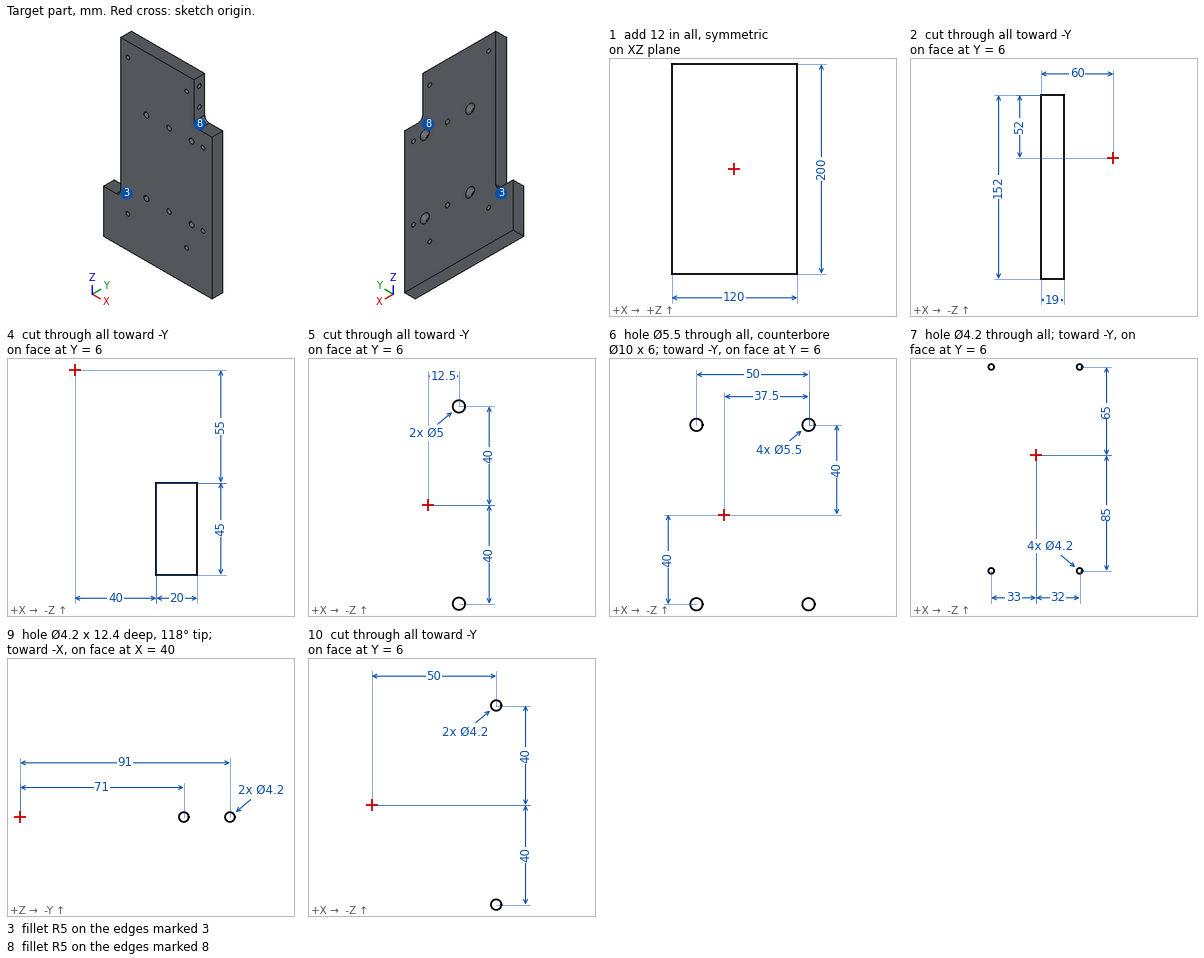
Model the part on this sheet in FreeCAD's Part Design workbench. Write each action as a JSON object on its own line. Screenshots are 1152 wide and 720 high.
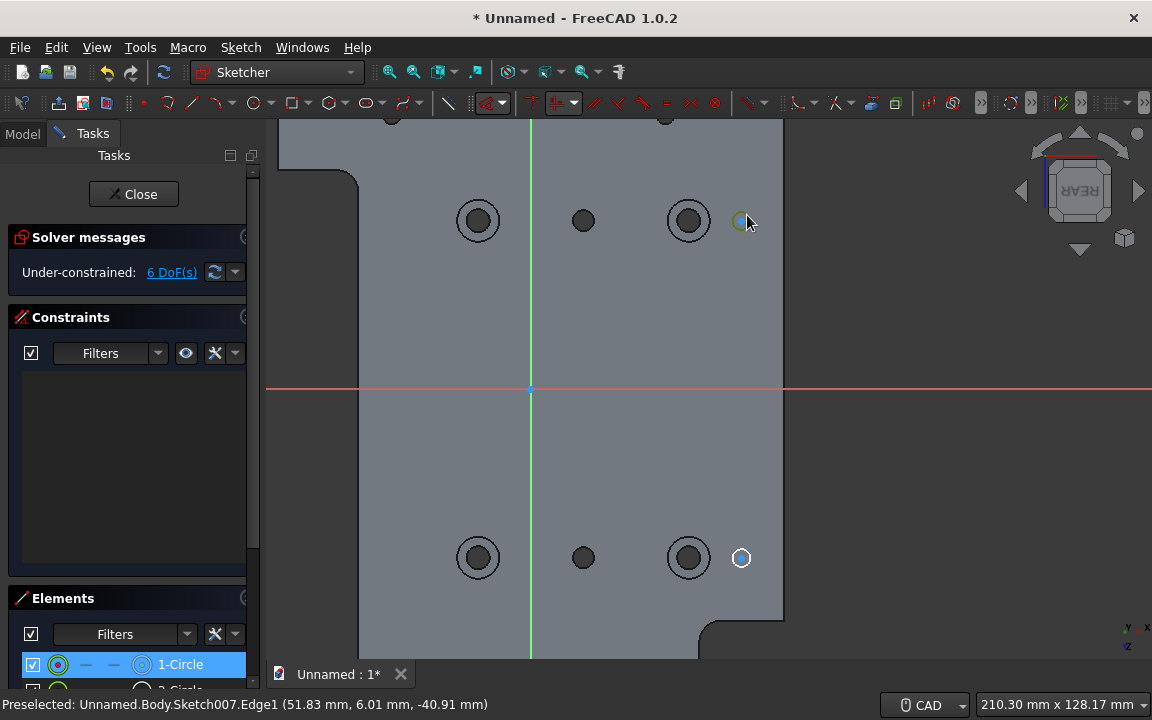
{"action": "scroll", "coordinate": [748, 552], "scroll_direction": "up", "scroll_amount": 3}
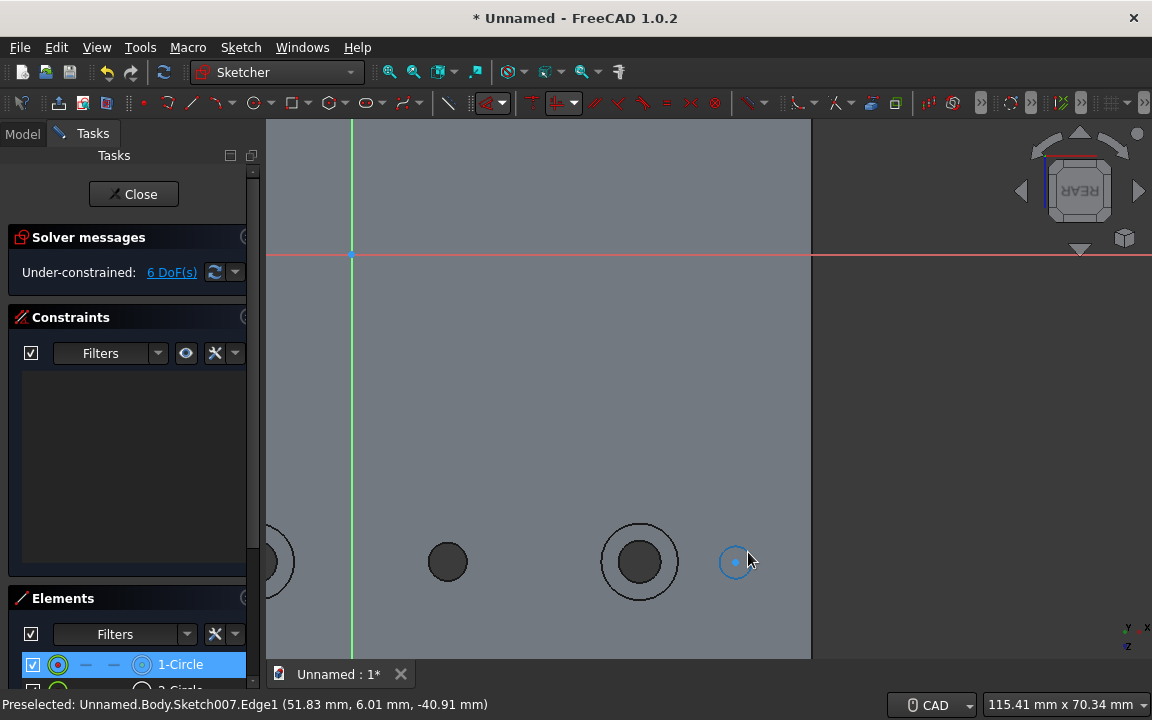
{"action": "left_click", "coordinate": [747, 551]}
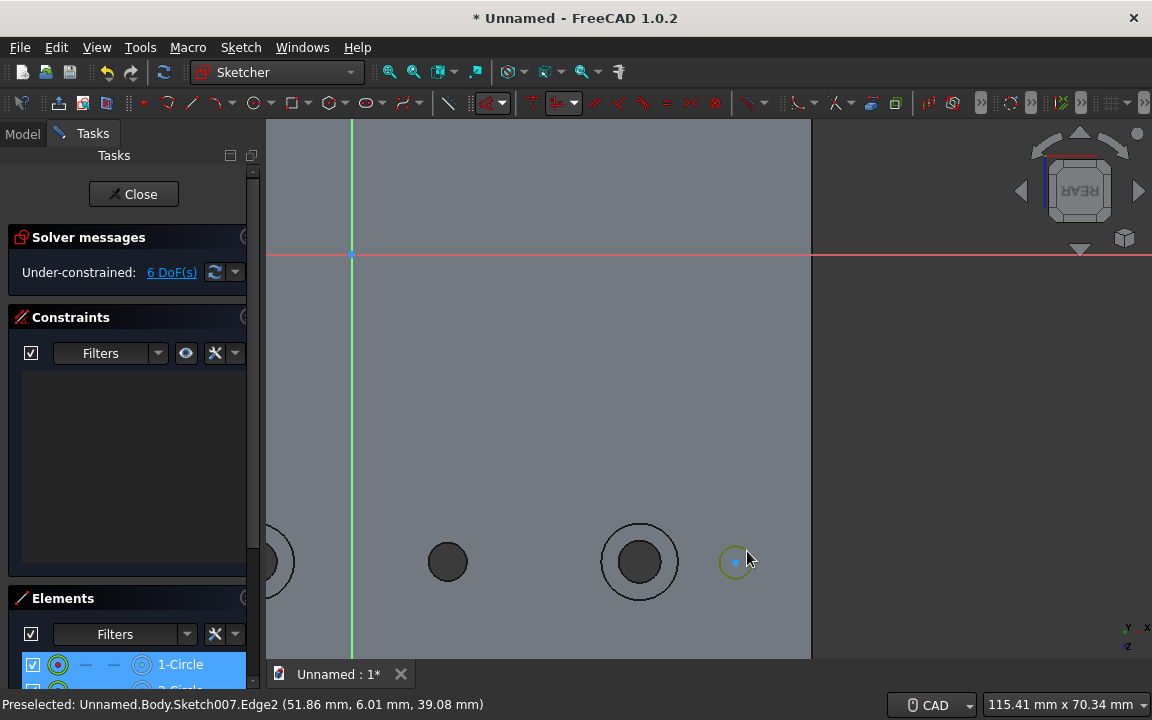
{"action": "left_click", "coordinate": [668, 104]}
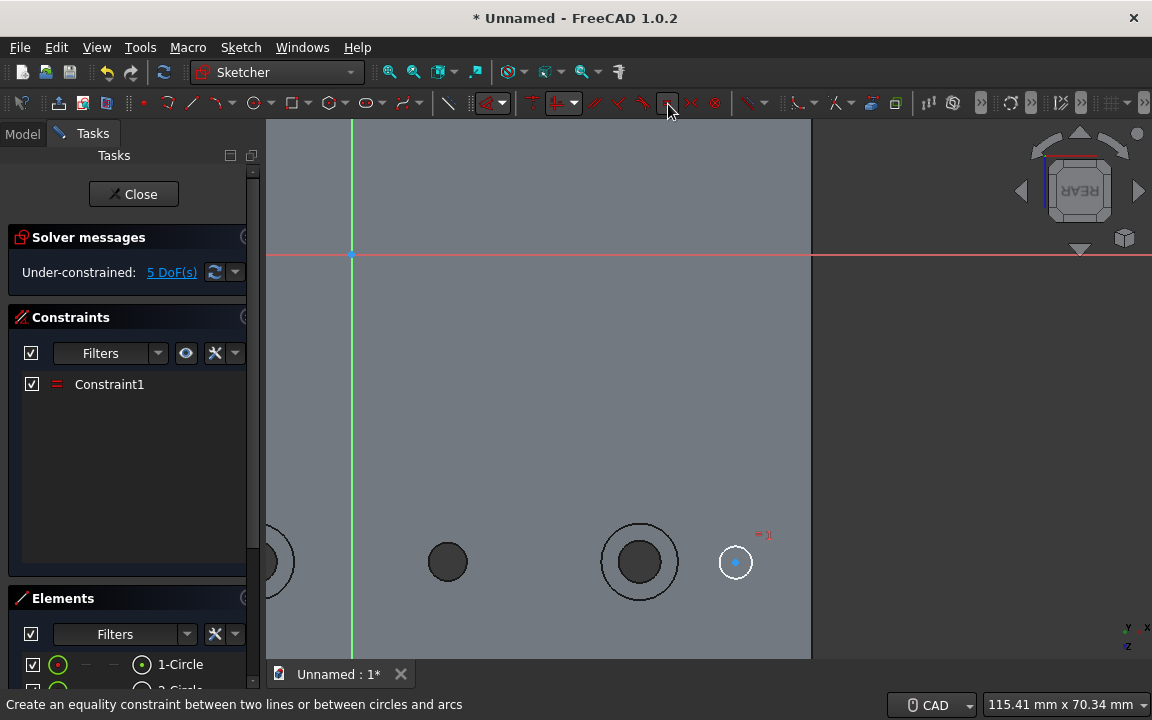
{"action": "scroll", "coordinate": [748, 552], "scroll_direction": "down", "scroll_amount": 3}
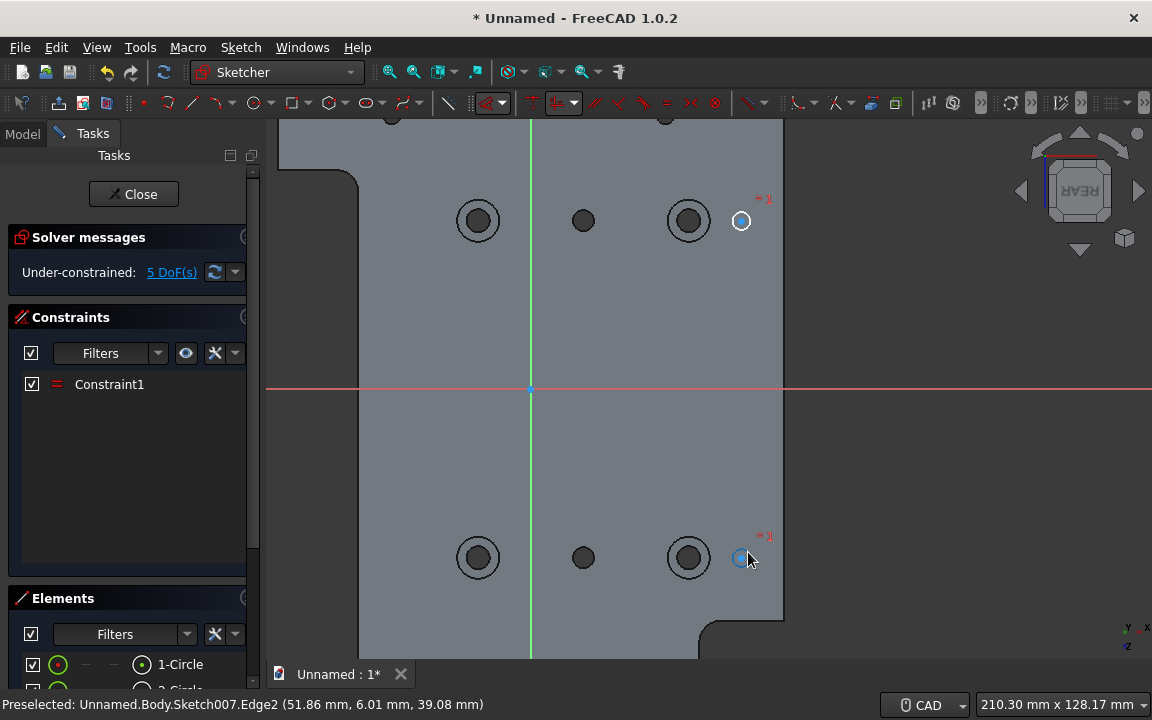
{"action": "left_click", "coordinate": [741, 221]}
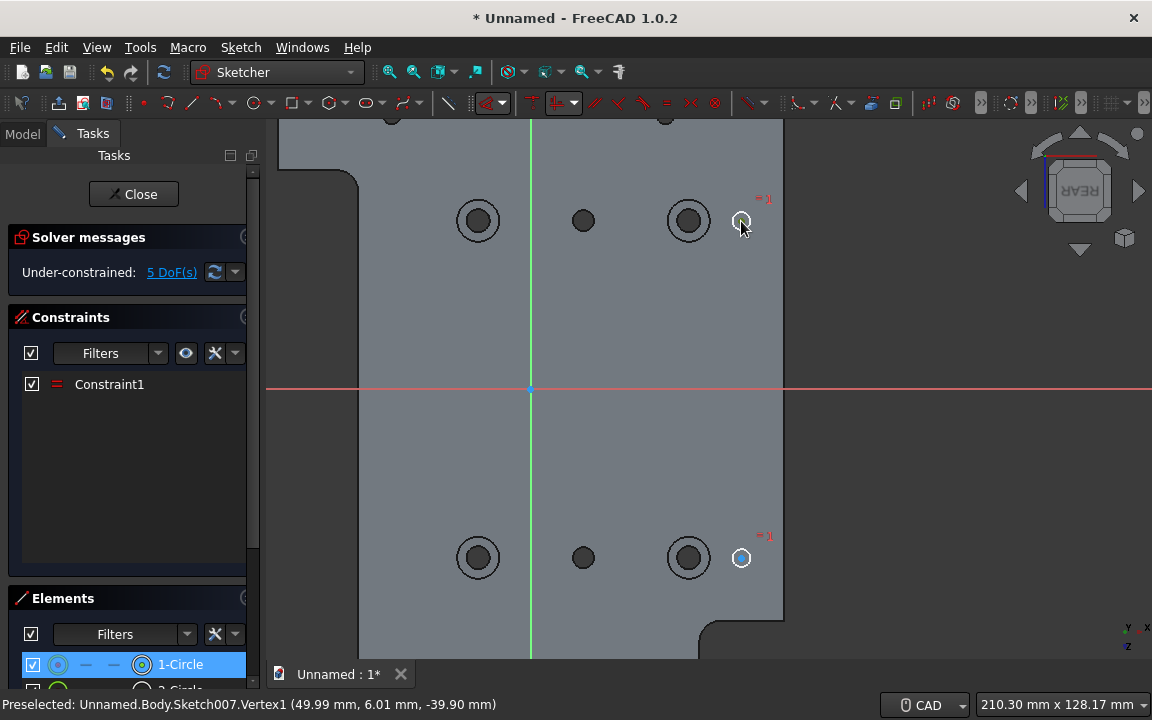
{"action": "left_click", "coordinate": [742, 558]}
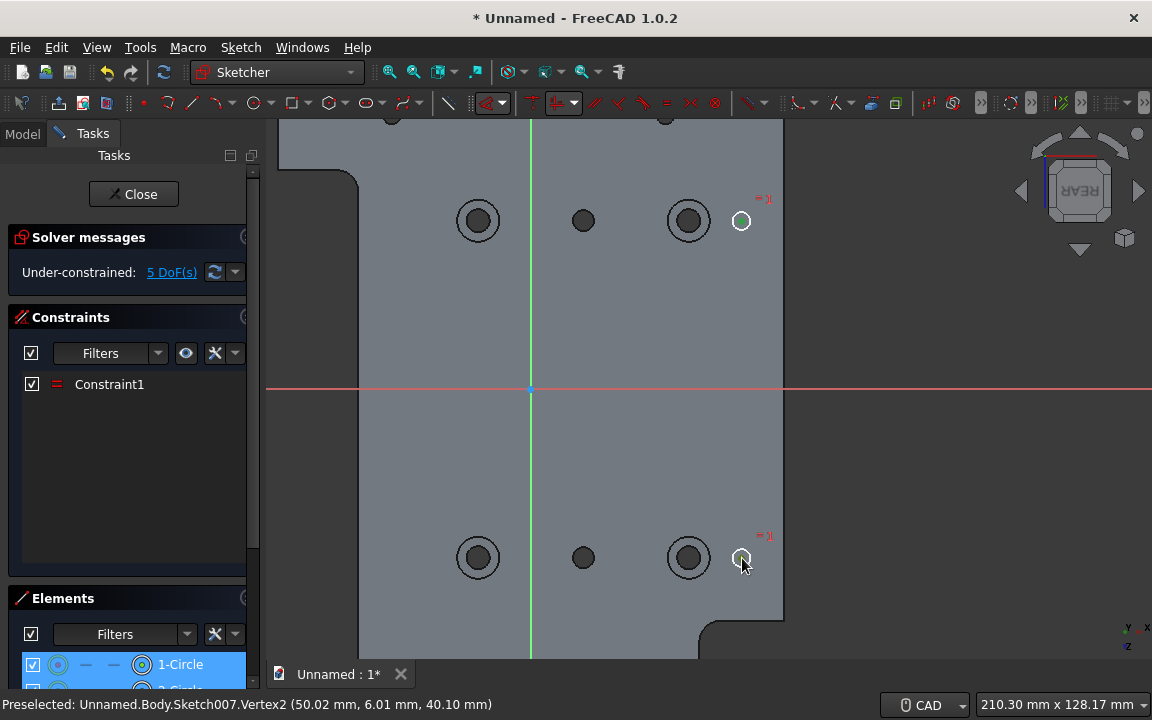
{"action": "key", "text": "v"}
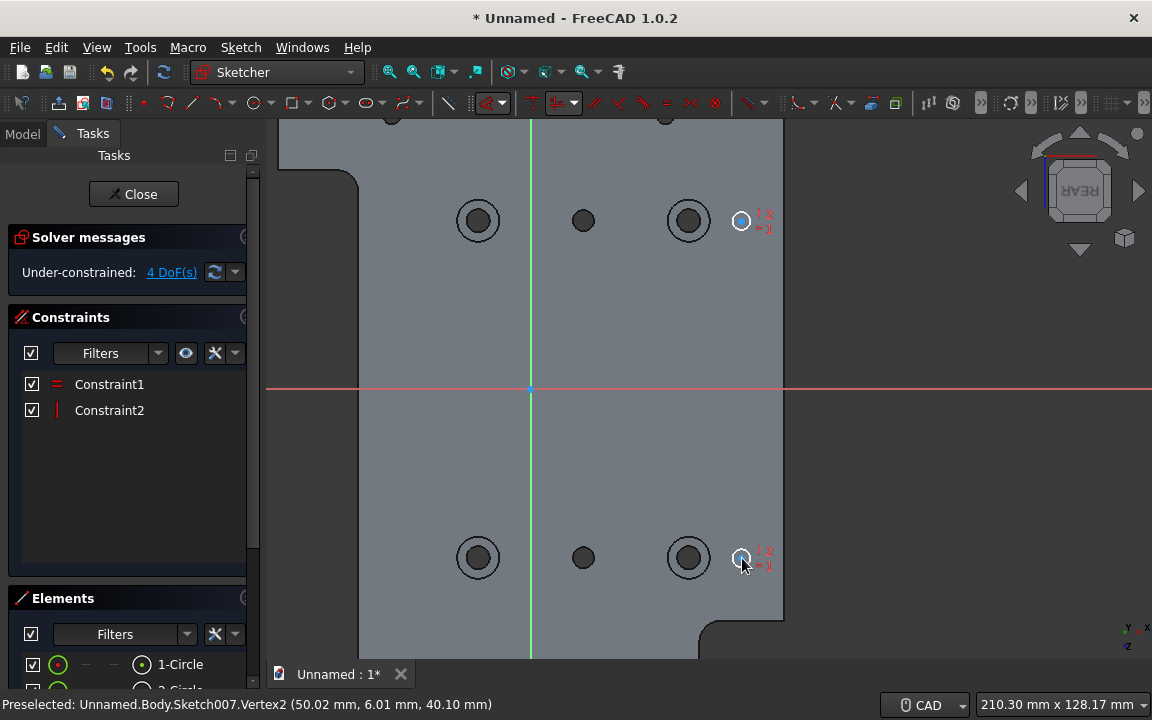
{"action": "scroll", "coordinate": [742, 212], "scroll_direction": "up", "scroll_amount": 5}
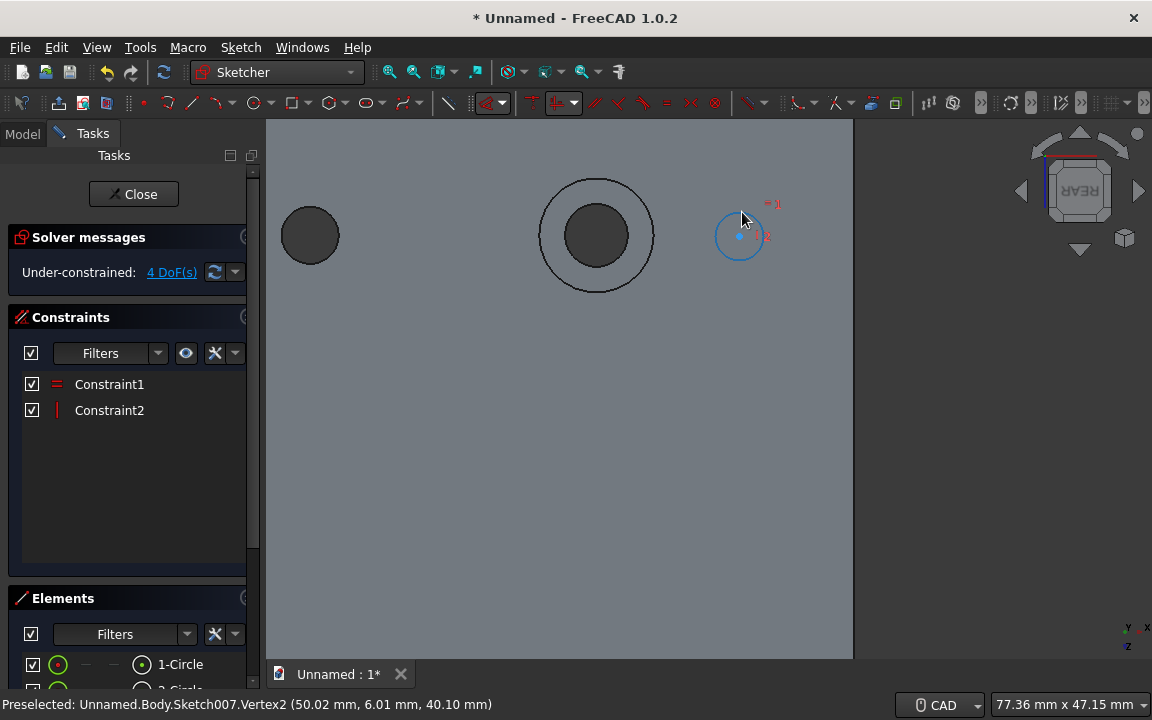
{"action": "left_click", "coordinate": [740, 212]}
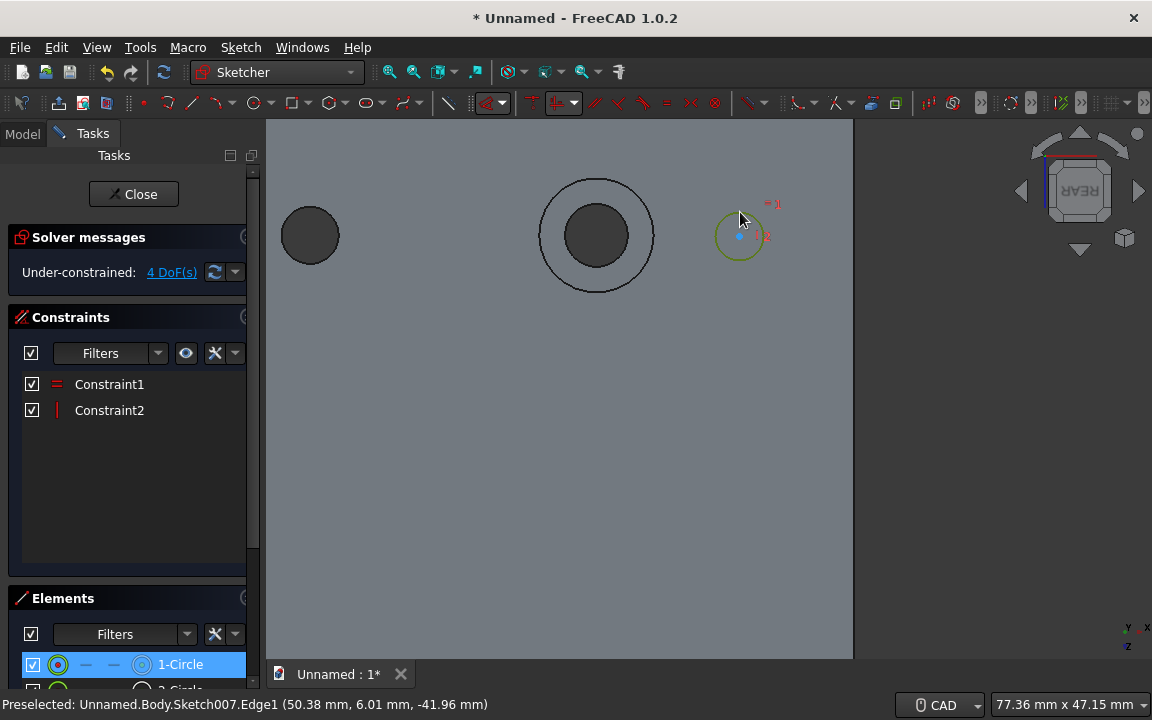
{"action": "left_click", "coordinate": [504, 104]}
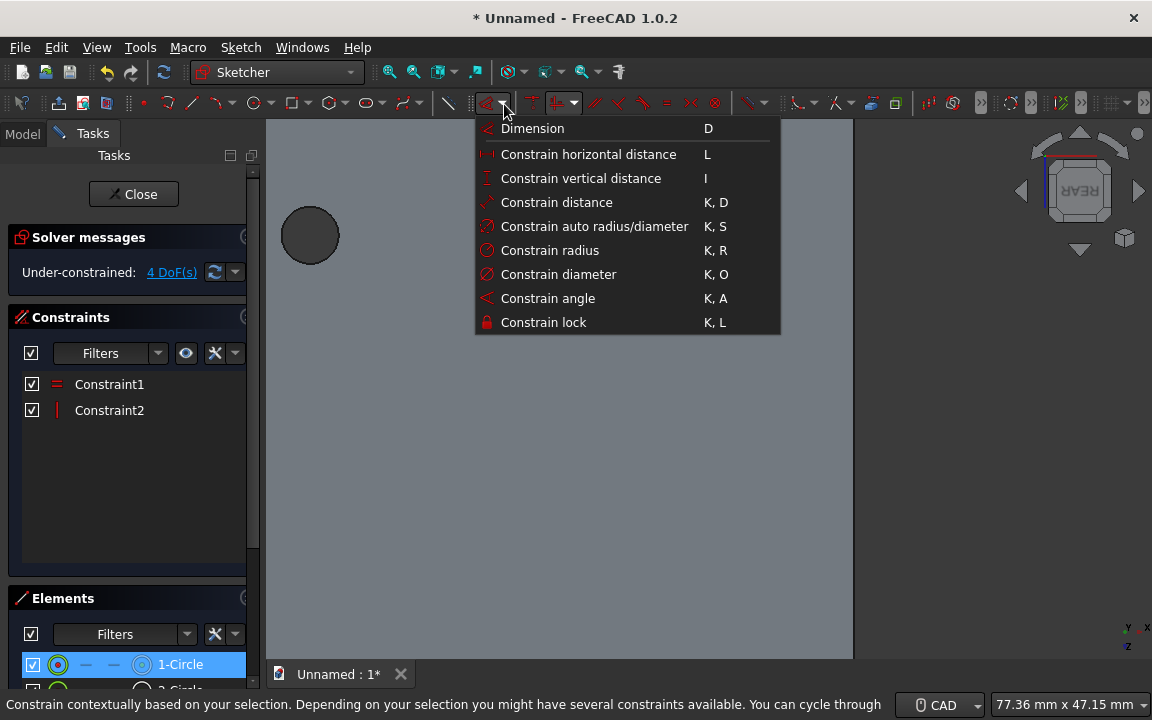
{"action": "left_click", "coordinate": [628, 274]}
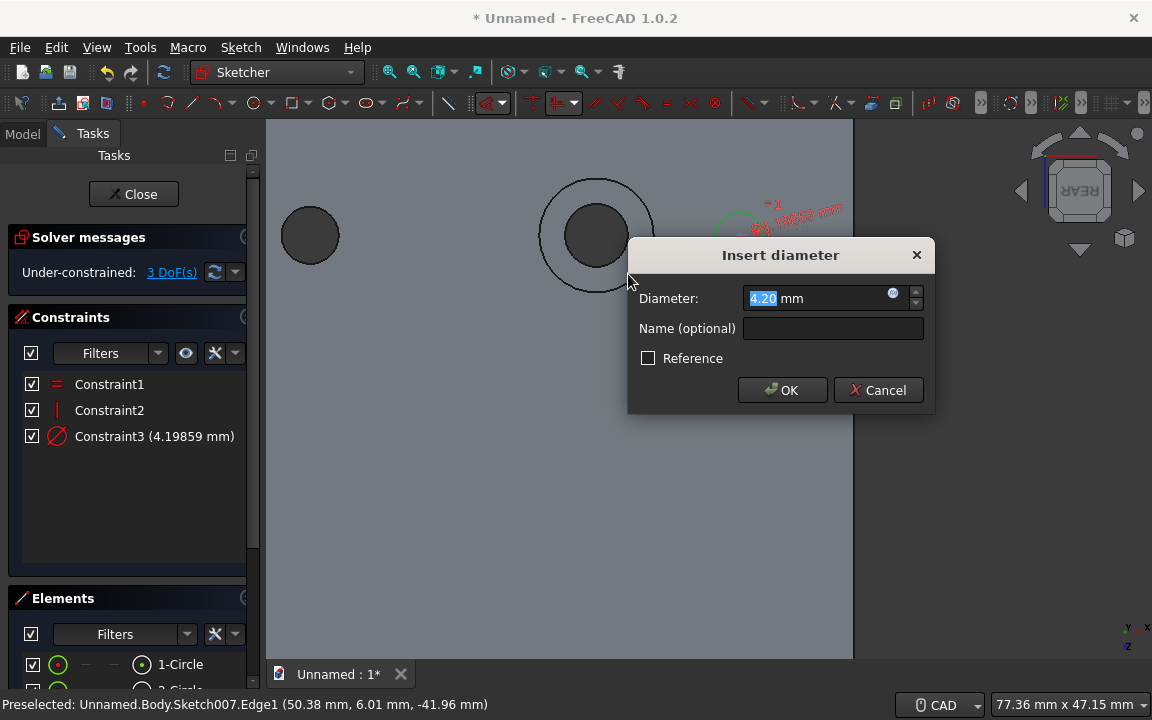
{"action": "type", "text": "4.2"}
{"action": "key", "text": "Return"}